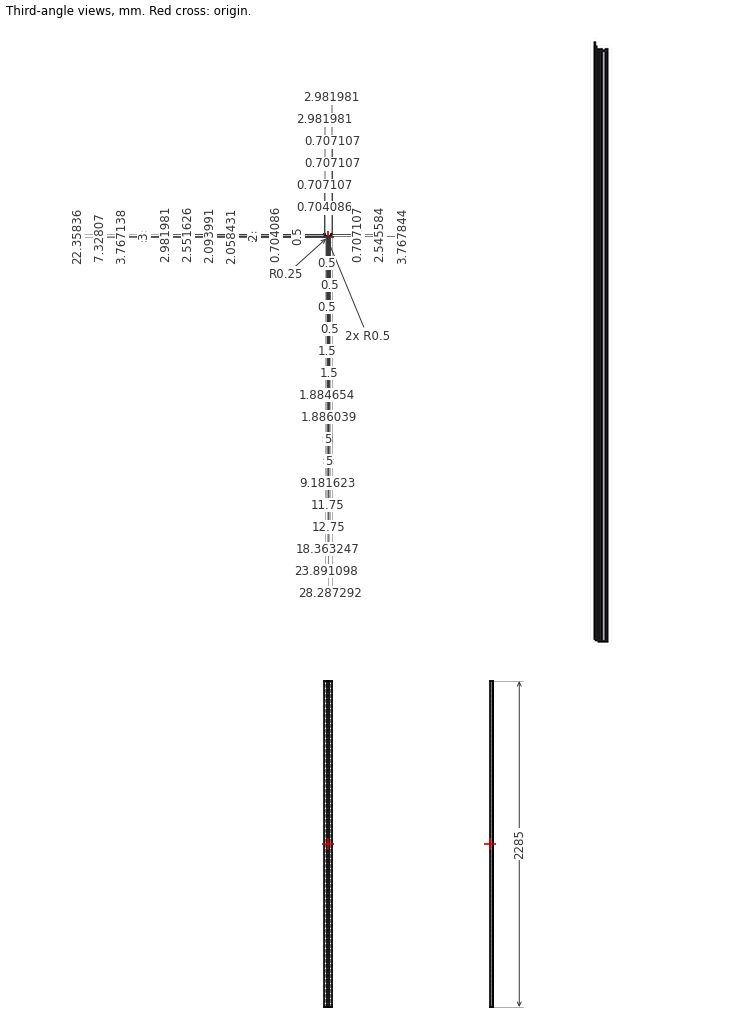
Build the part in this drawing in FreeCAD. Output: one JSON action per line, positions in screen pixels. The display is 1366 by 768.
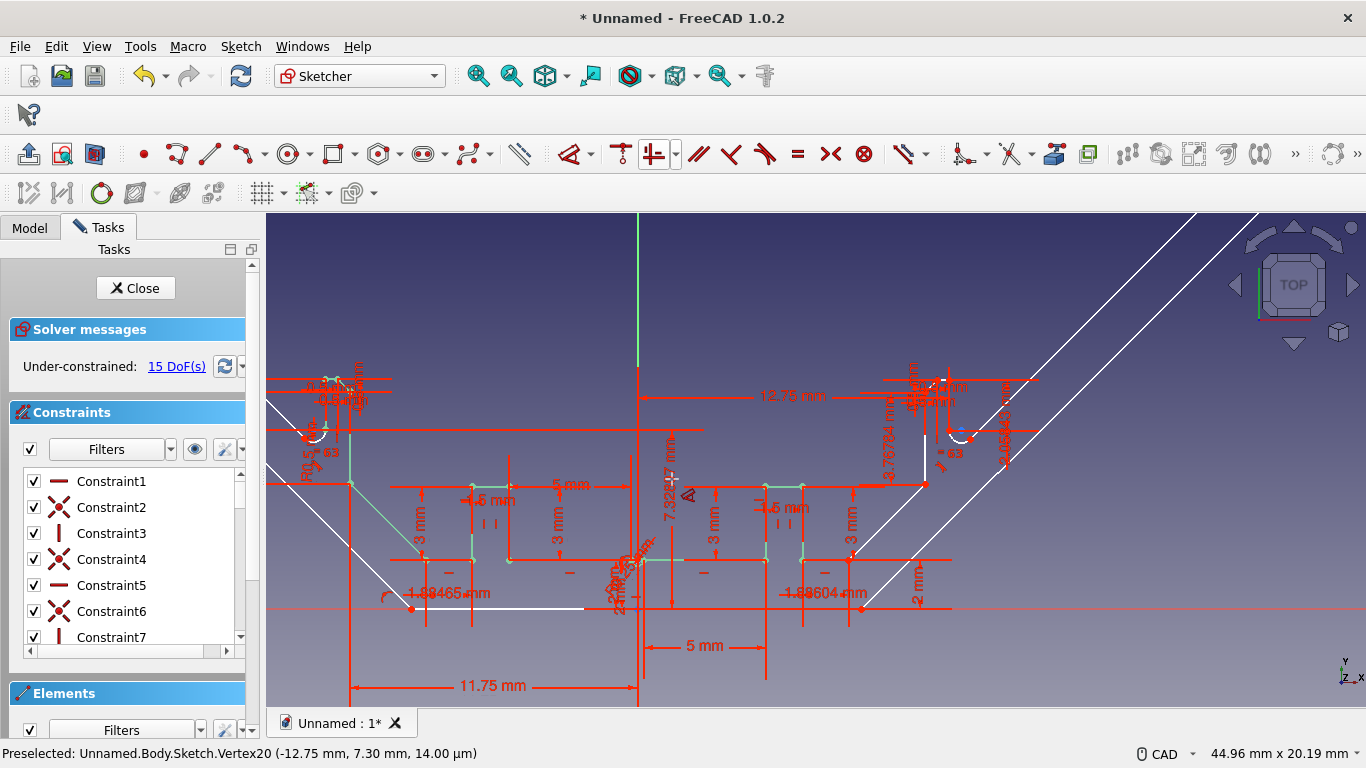
{"action": "left_click", "coordinate": [949, 431]}
{"action": "left_click", "coordinate": [983, 520]}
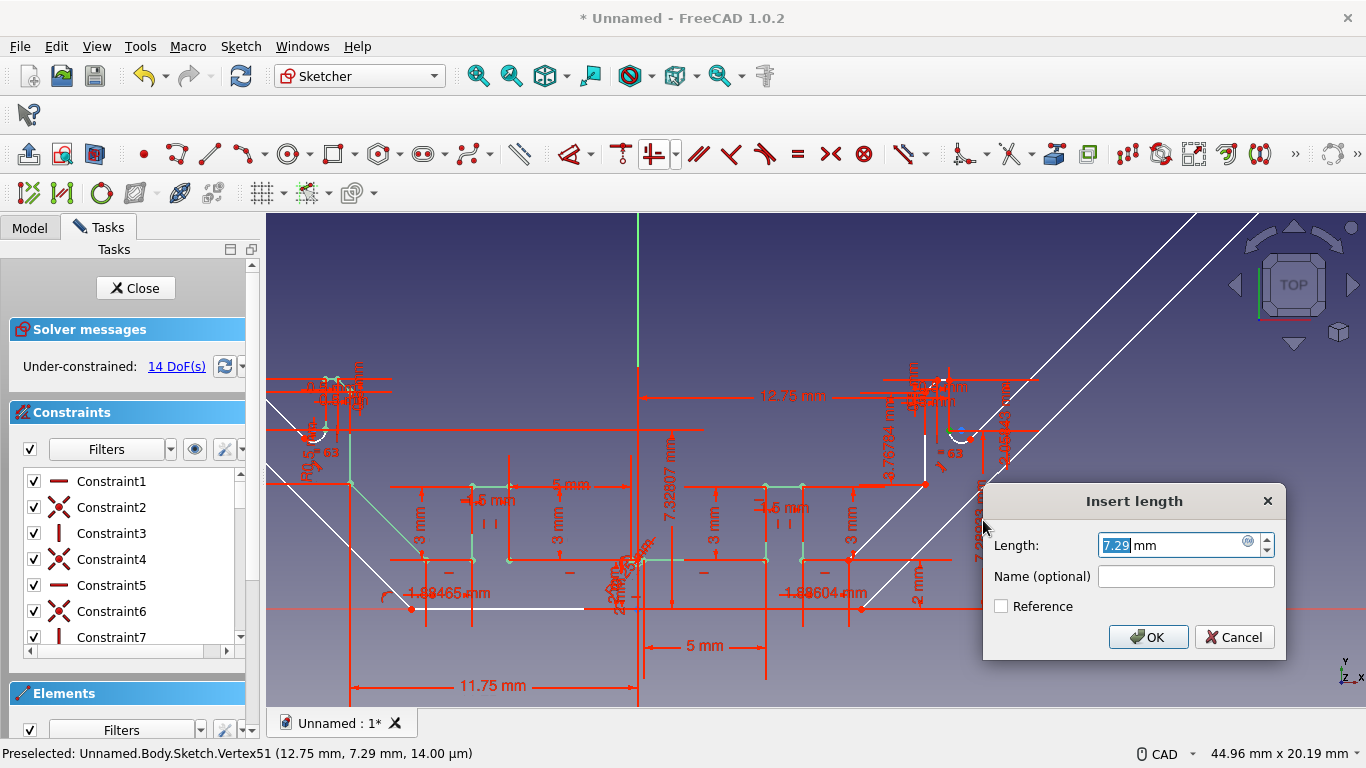
{"action": "type", "text": "7.32807"}
{"action": "key", "text": "Return"}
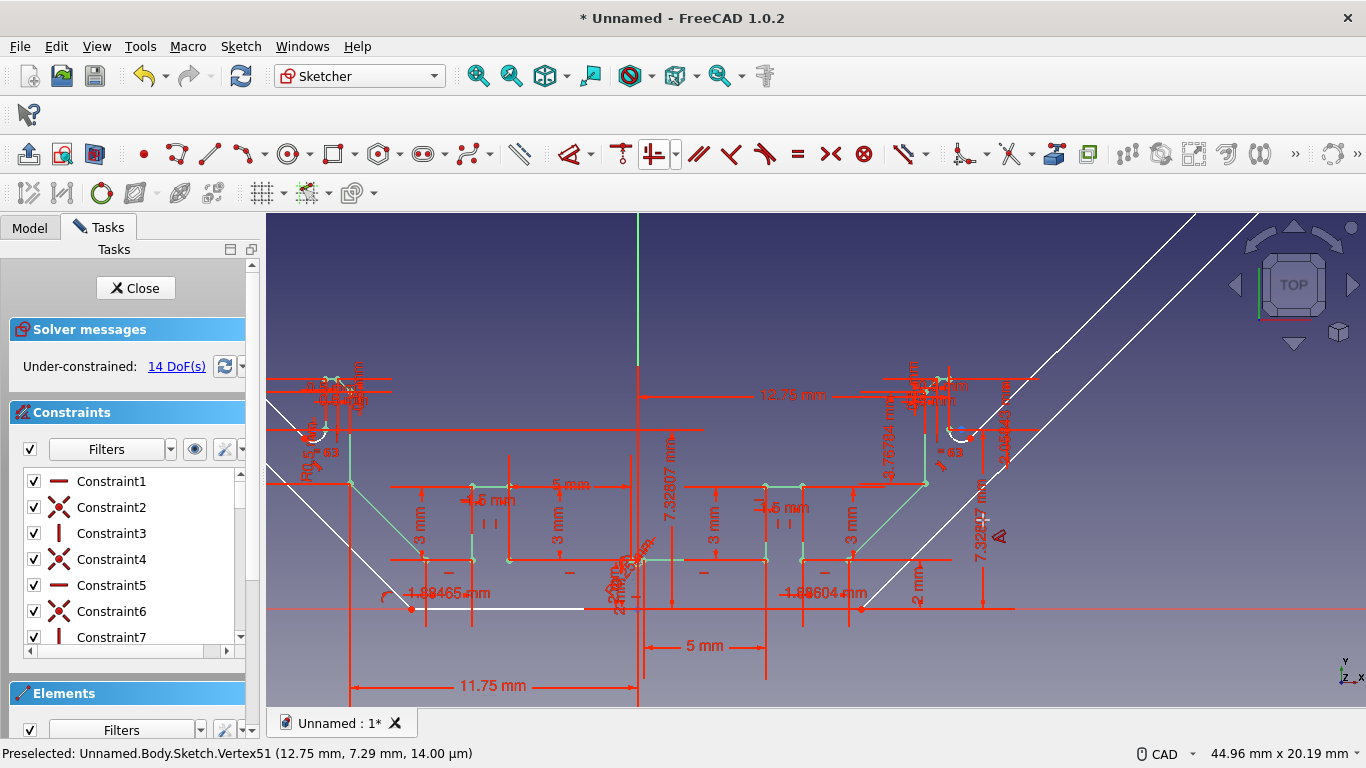
{"action": "left_click", "coordinate": [547, 609]}
{"action": "left_click", "coordinate": [533, 643]}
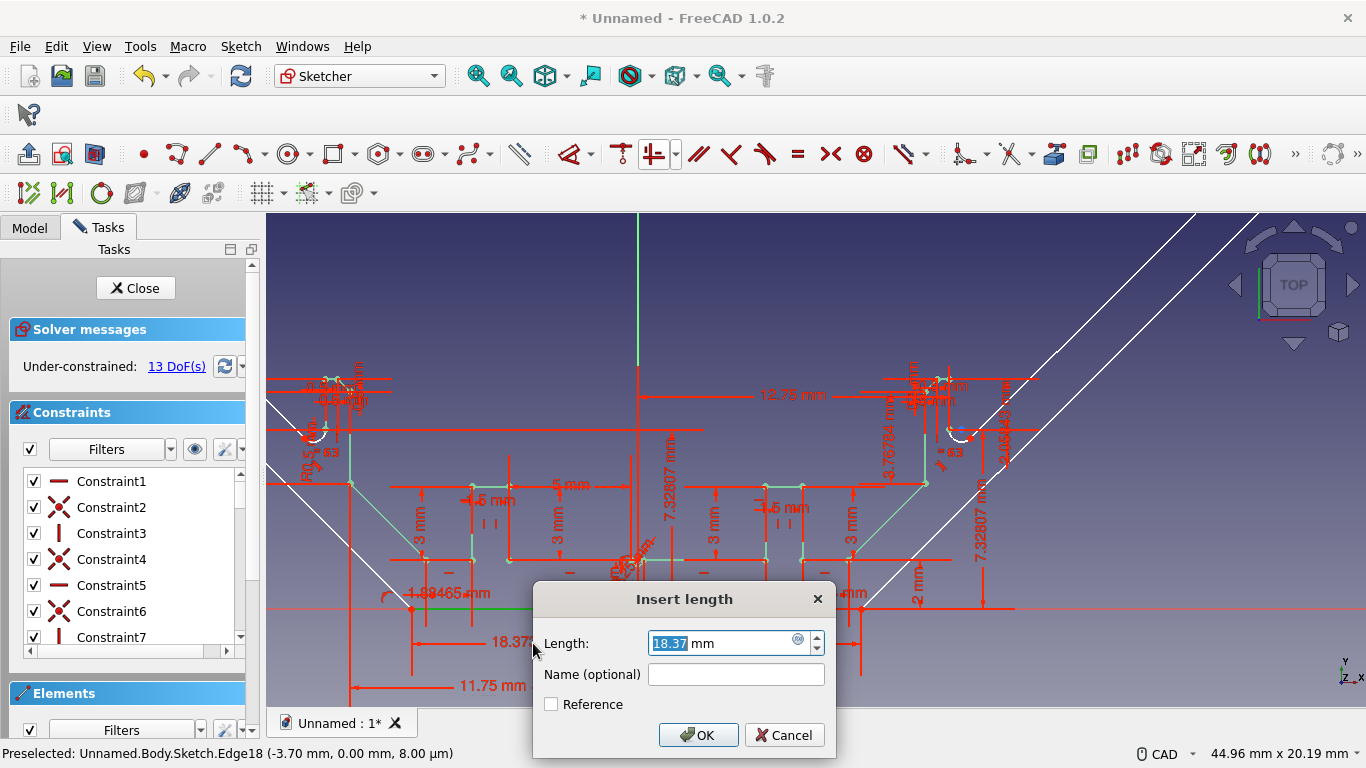
{"action": "type", "text": "18.363247"}
{"action": "key", "text": "Return"}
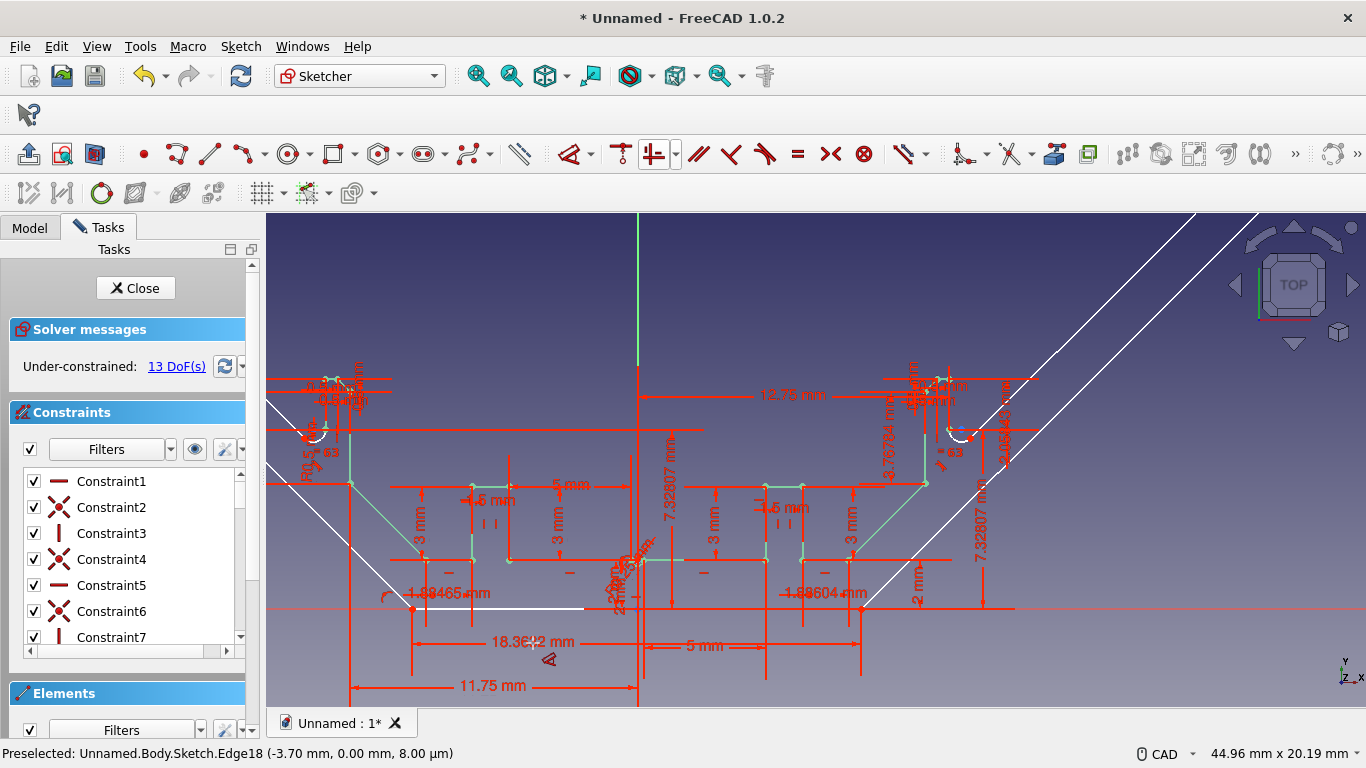
{"action": "scroll", "coordinate": [837, 562], "scroll_direction": "down", "scroll_amount": 4}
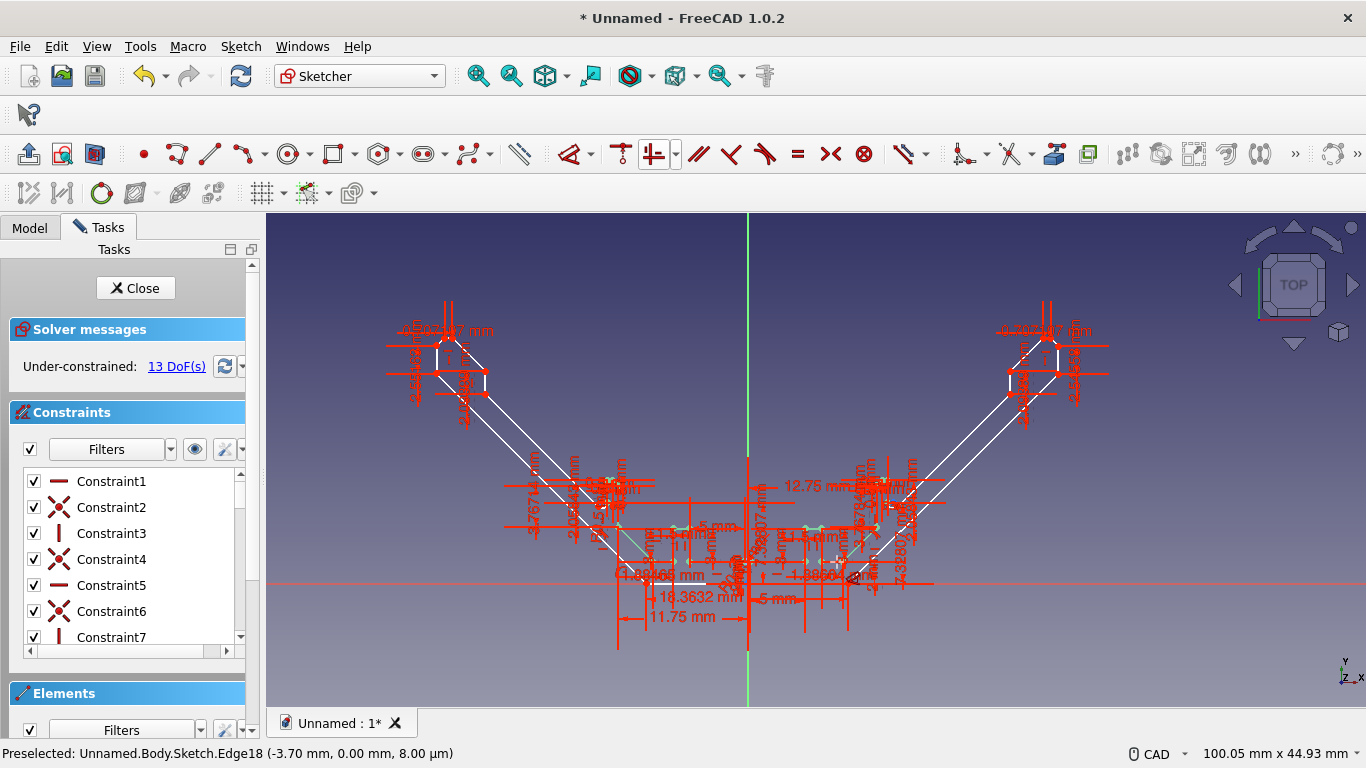
{"action": "scroll", "coordinate": [452, 338], "scroll_direction": "up", "scroll_amount": 3}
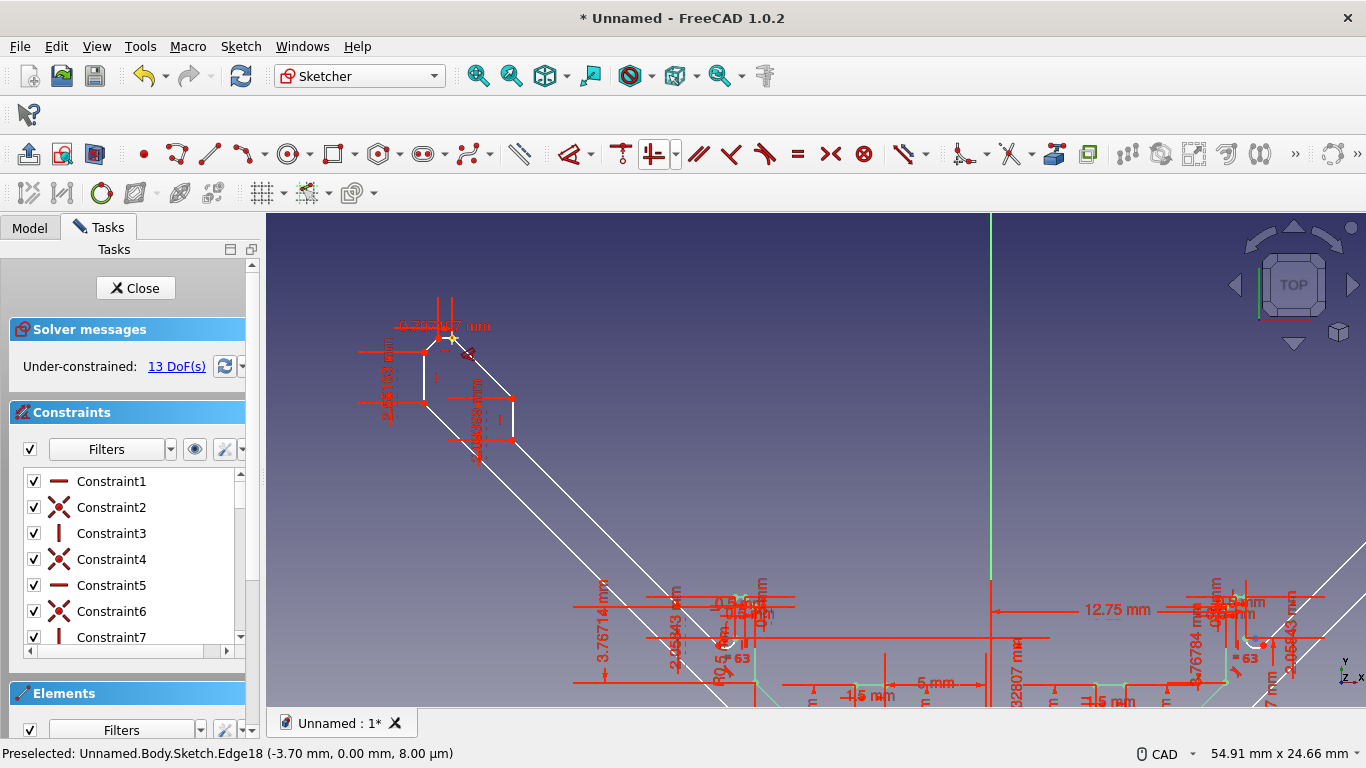
{"action": "left_click", "coordinate": [452, 338]}
{"action": "left_click", "coordinate": [418, 509]}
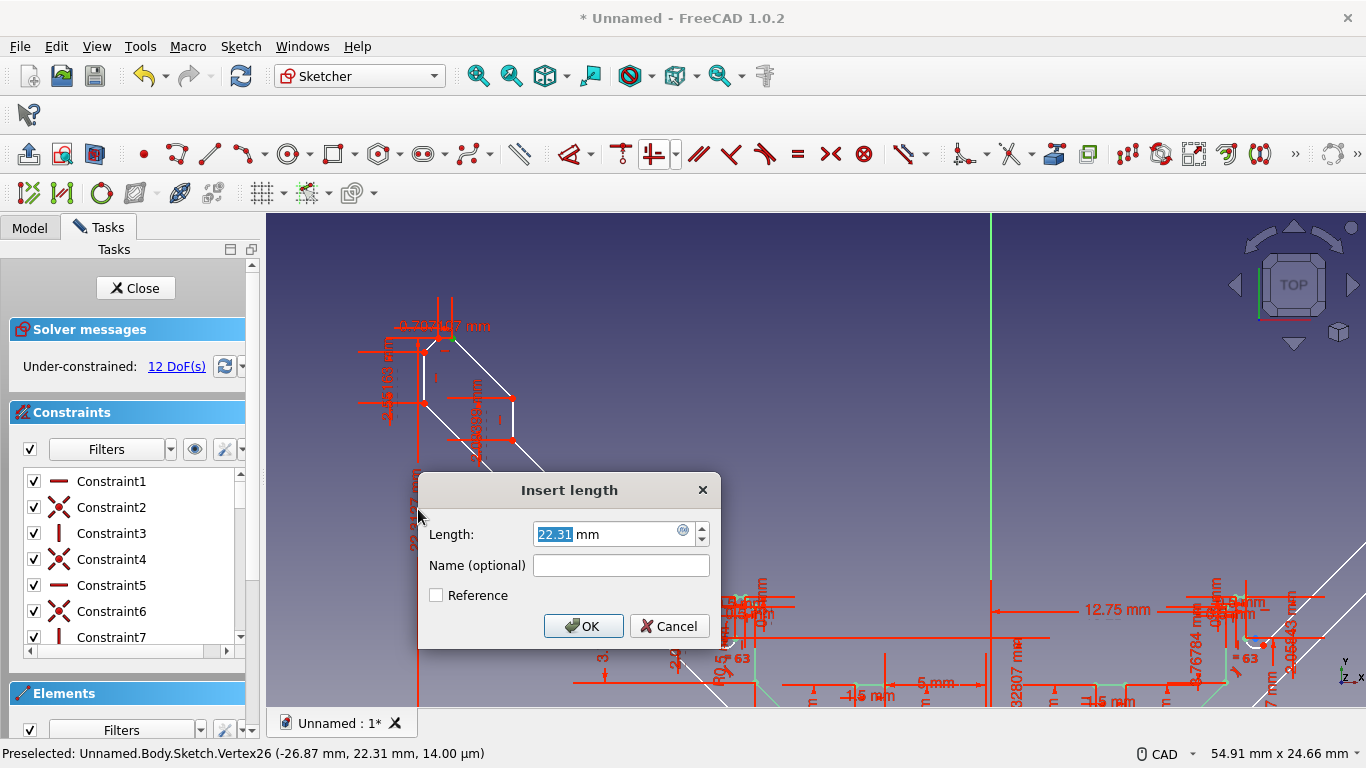
{"action": "type", "text": "22.35836"}
{"action": "key", "text": "Return"}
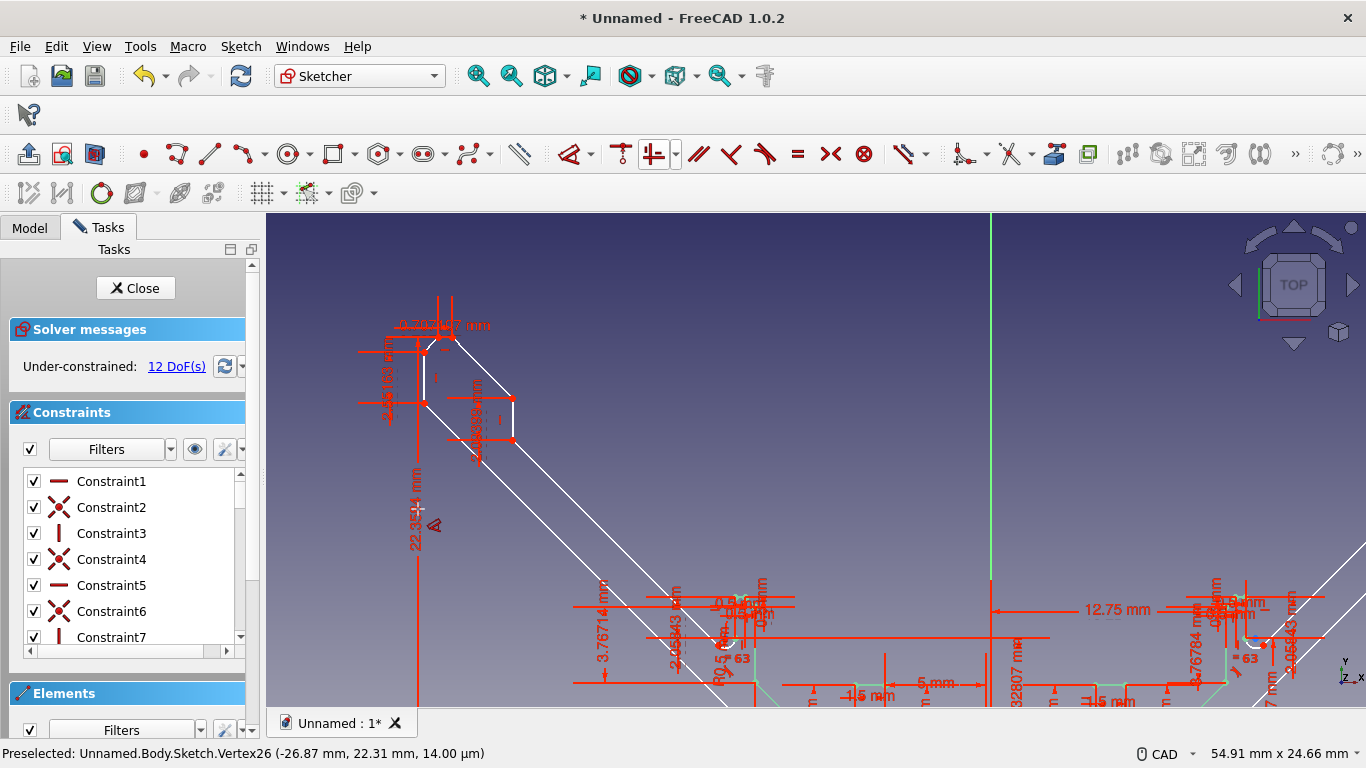
{"action": "scroll", "coordinate": [452, 337], "scroll_direction": "down", "scroll_amount": 3}